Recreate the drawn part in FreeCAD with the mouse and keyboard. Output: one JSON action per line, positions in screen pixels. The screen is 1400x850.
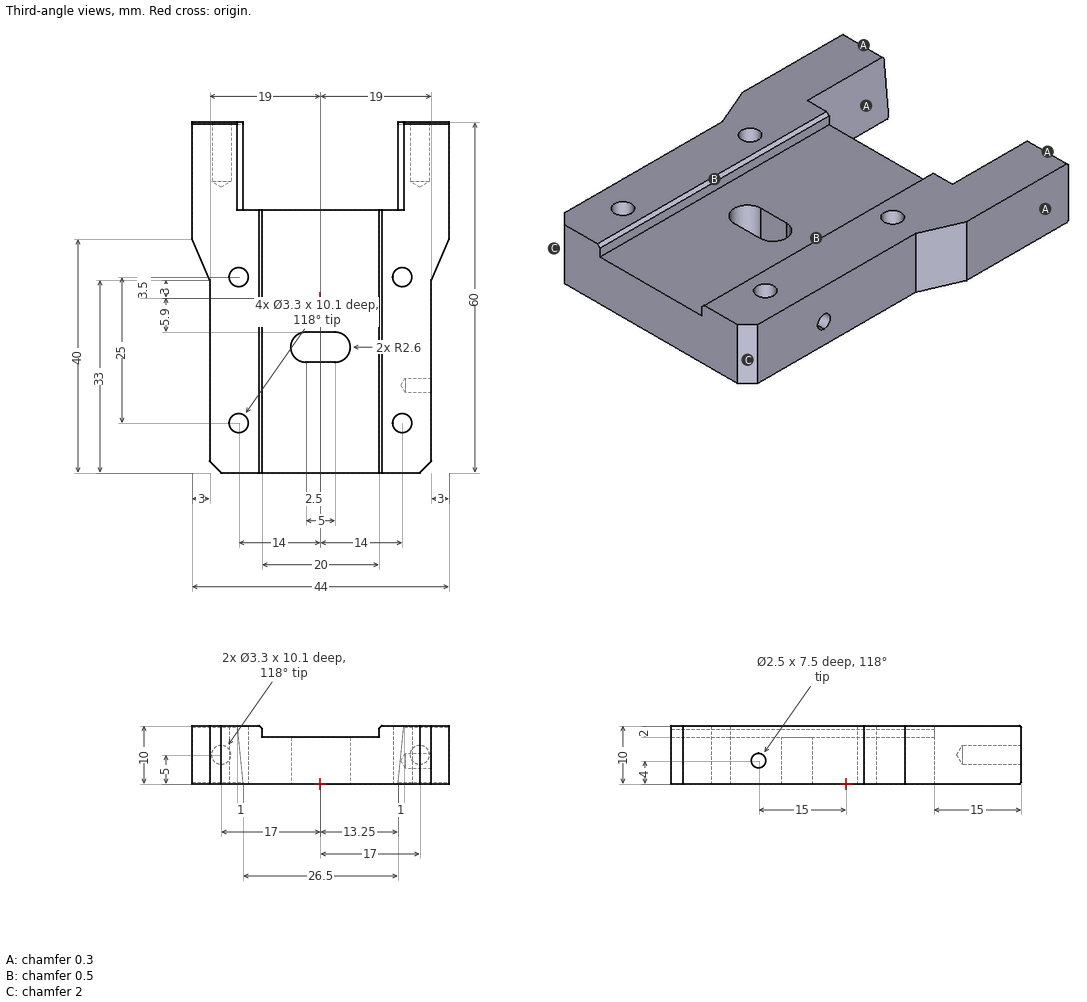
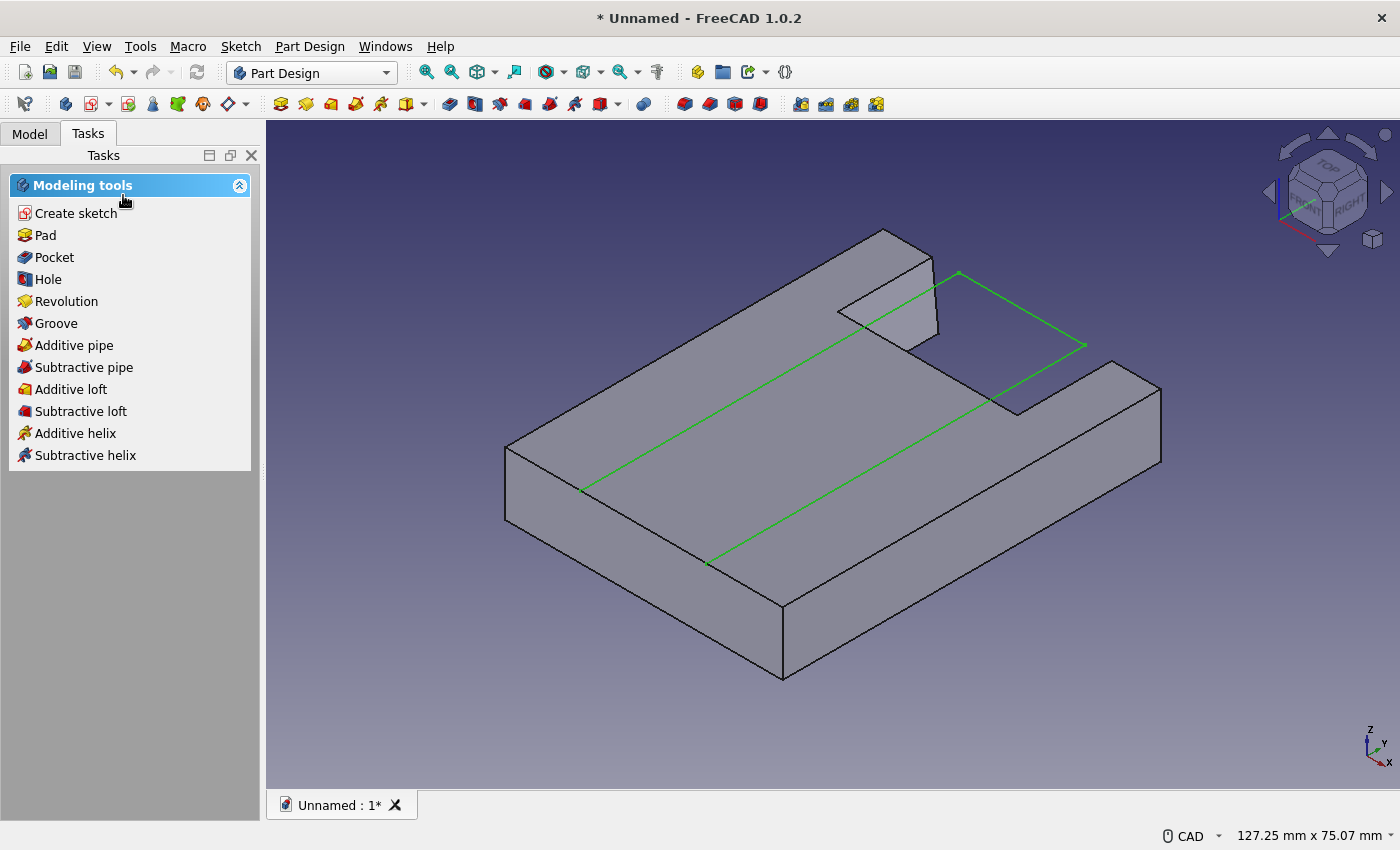
{"action": "left_click", "coordinate": [450, 104]}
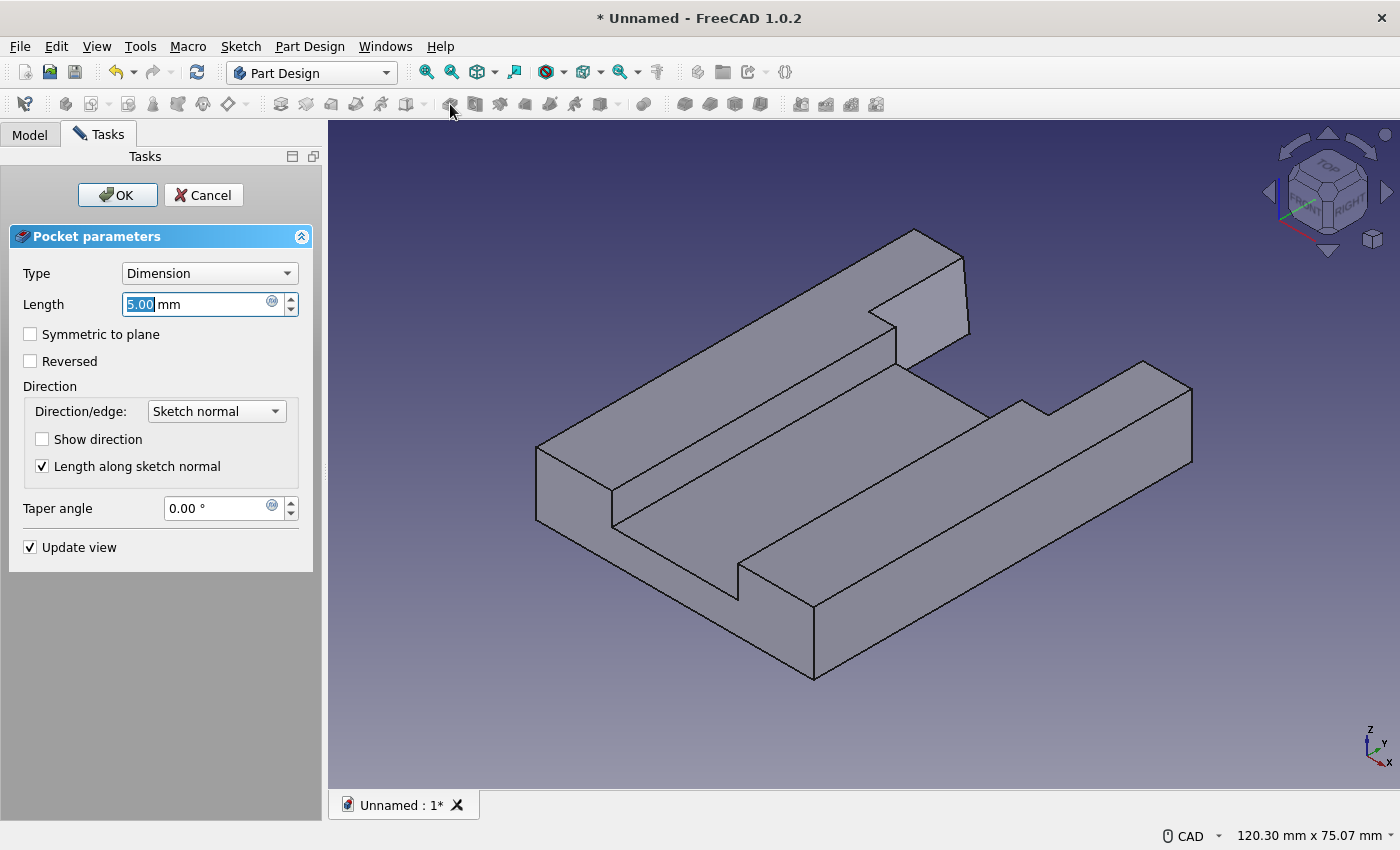
{"action": "type", "text": "2"}
{"action": "key", "text": "Tab"}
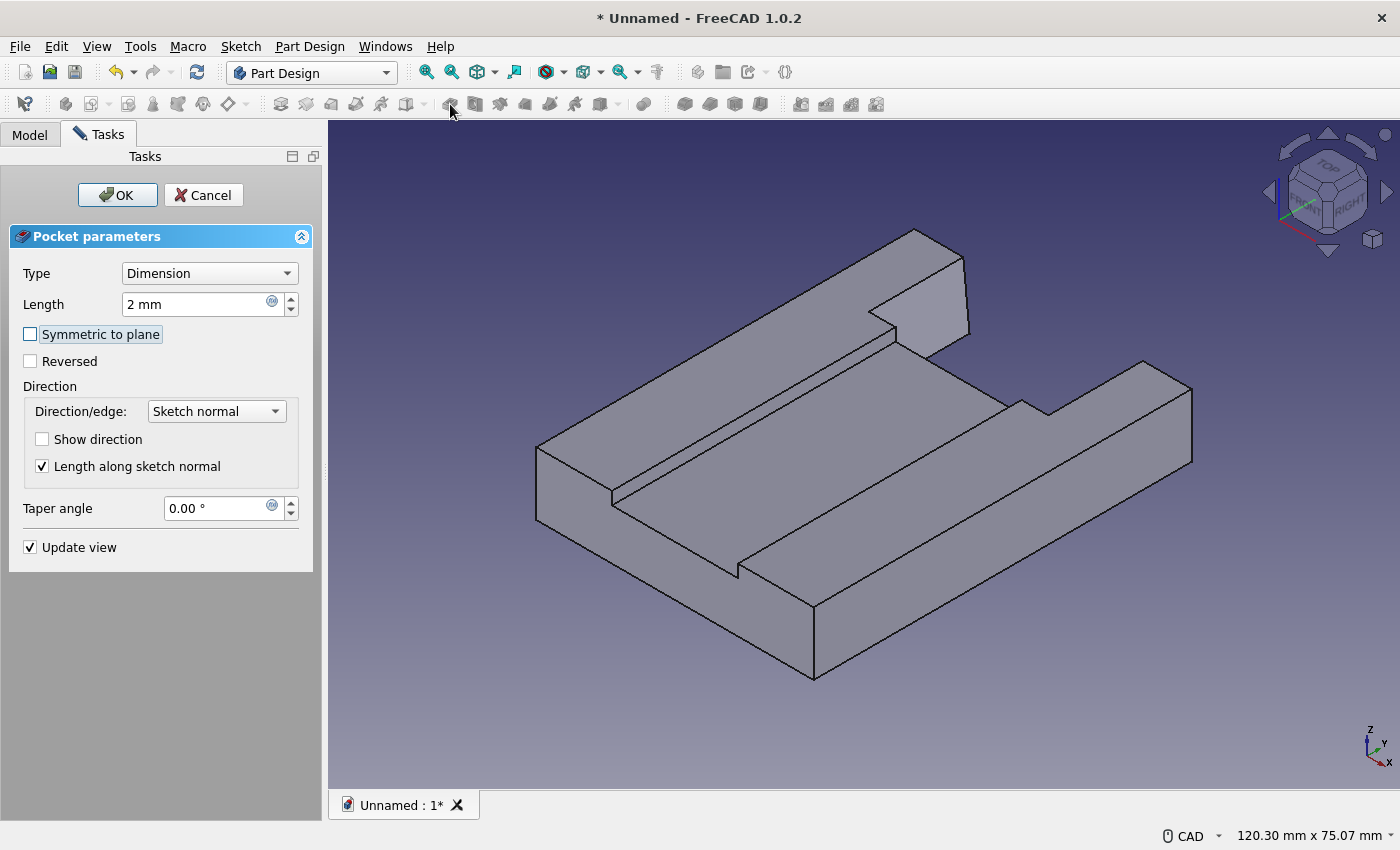
{"action": "left_click", "coordinate": [118, 195]}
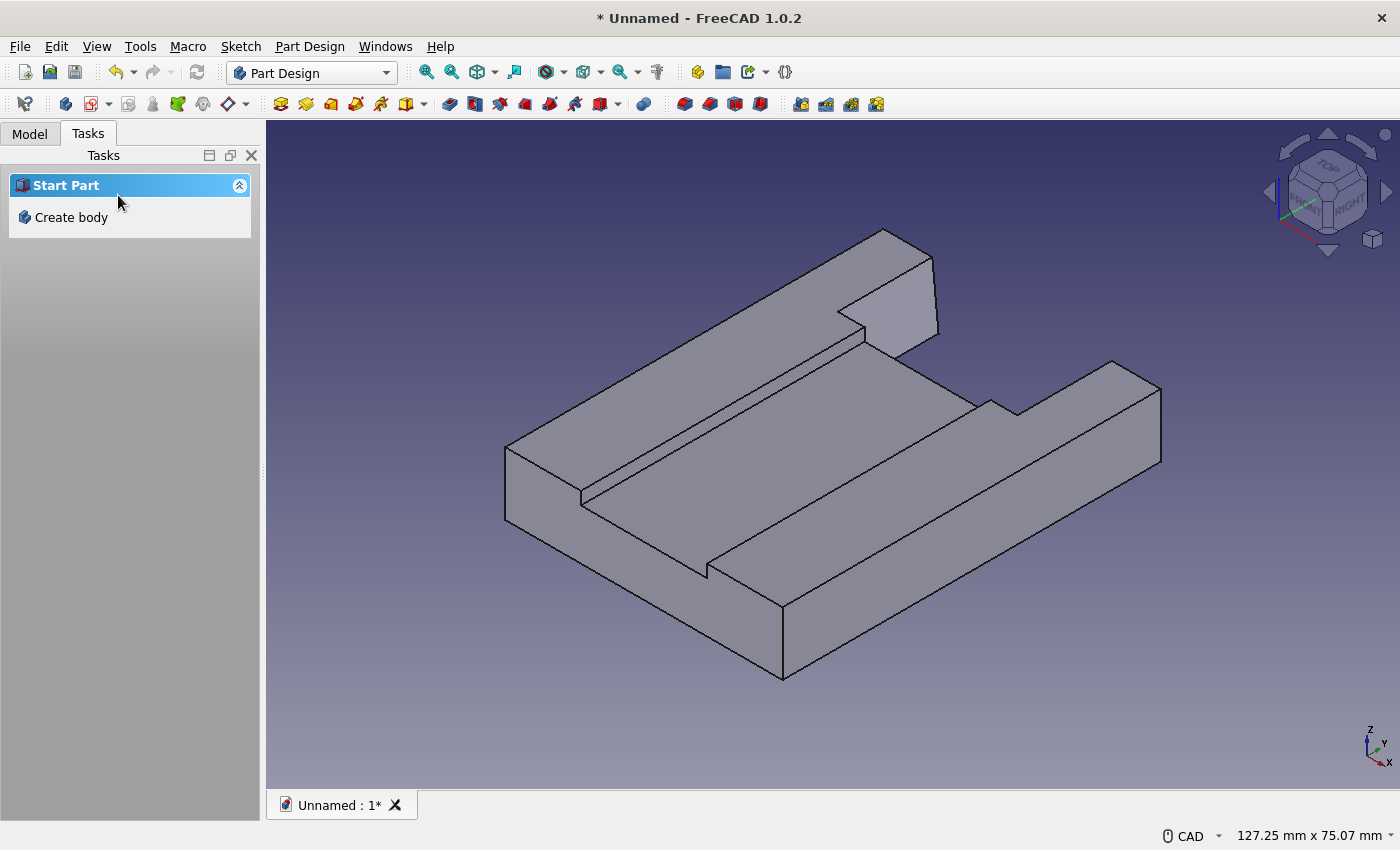
{"action": "key", "text": "4"}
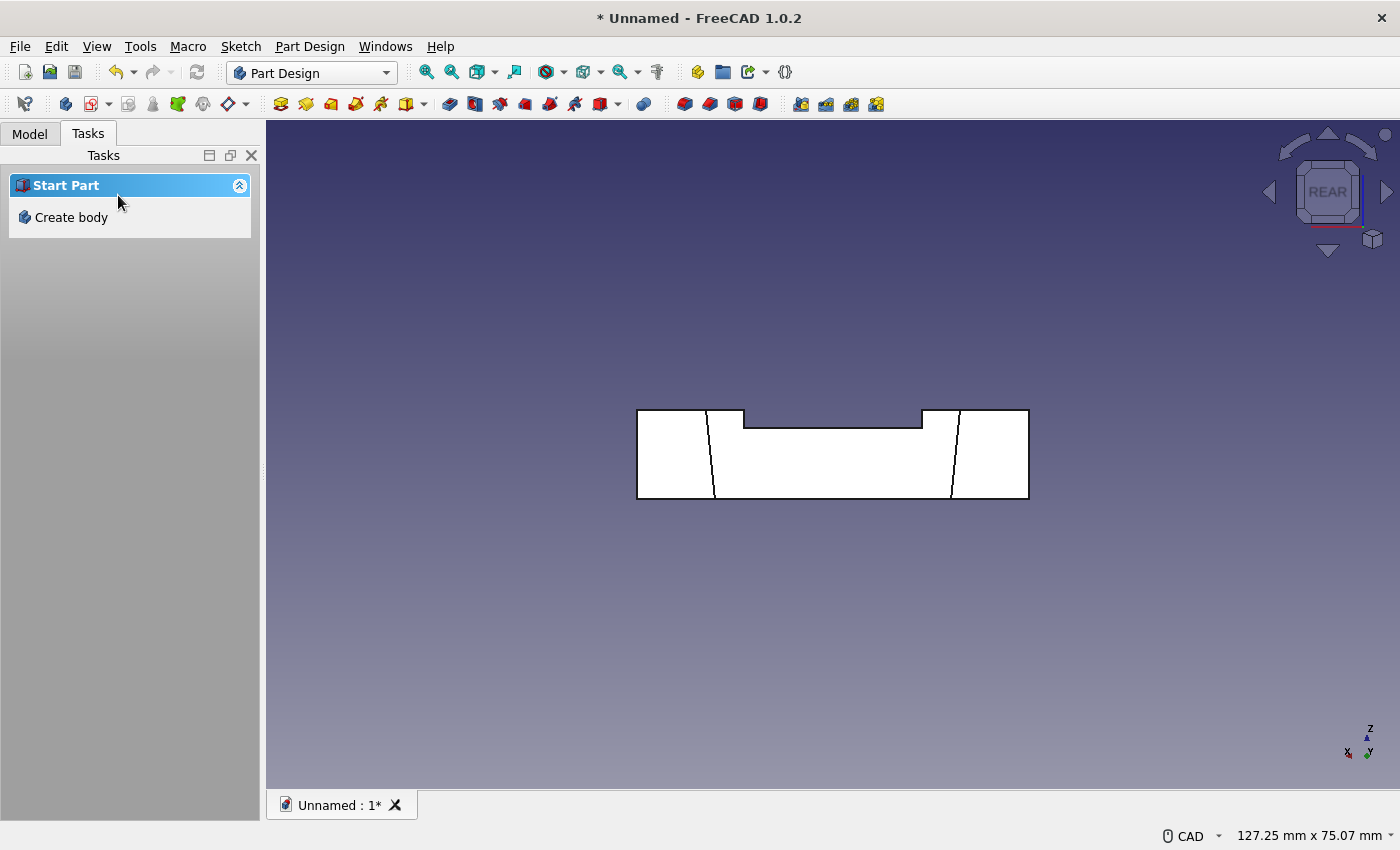
{"action": "left_click", "coordinate": [427, 72]}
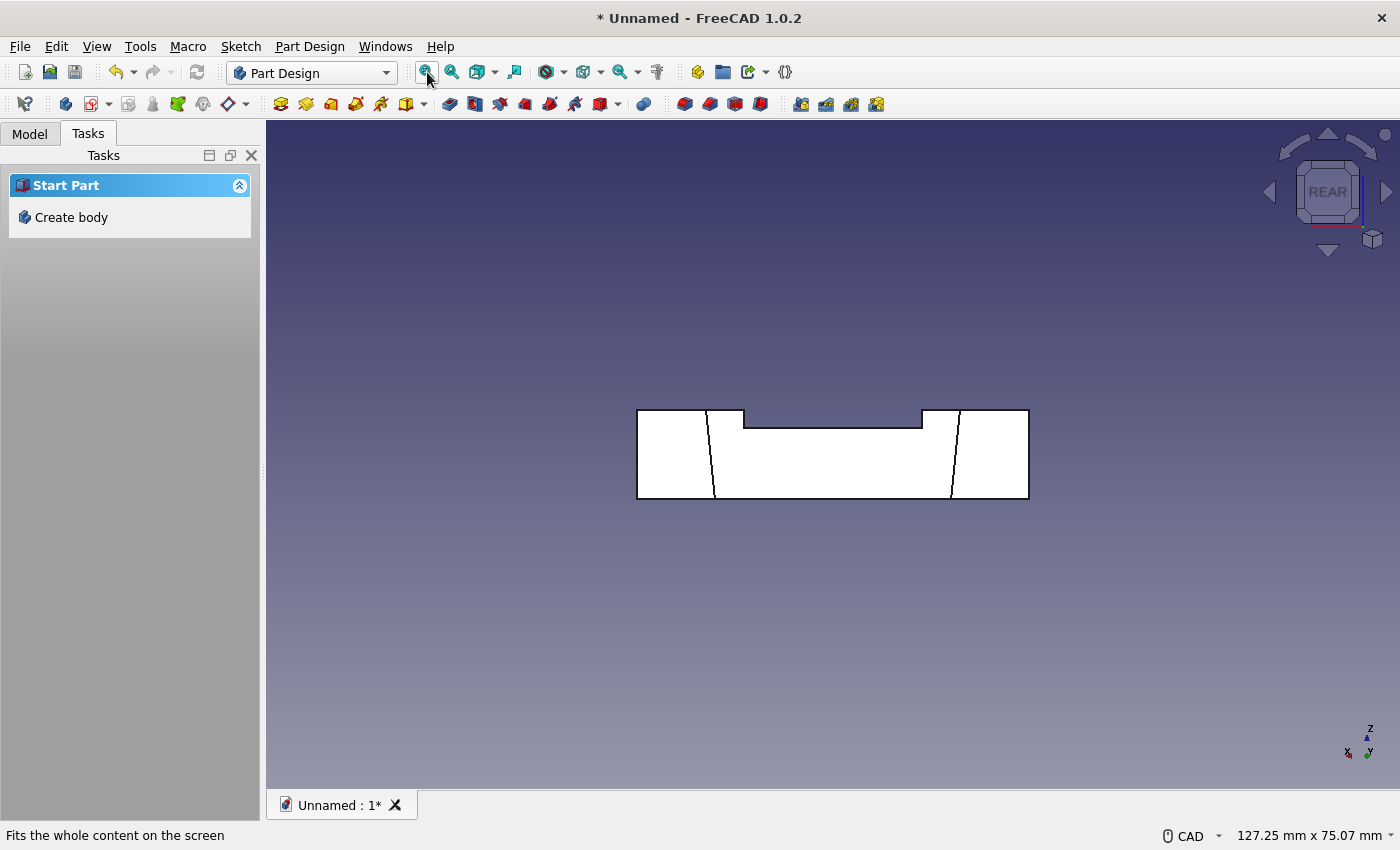
{"action": "left_click", "coordinate": [676, 454]}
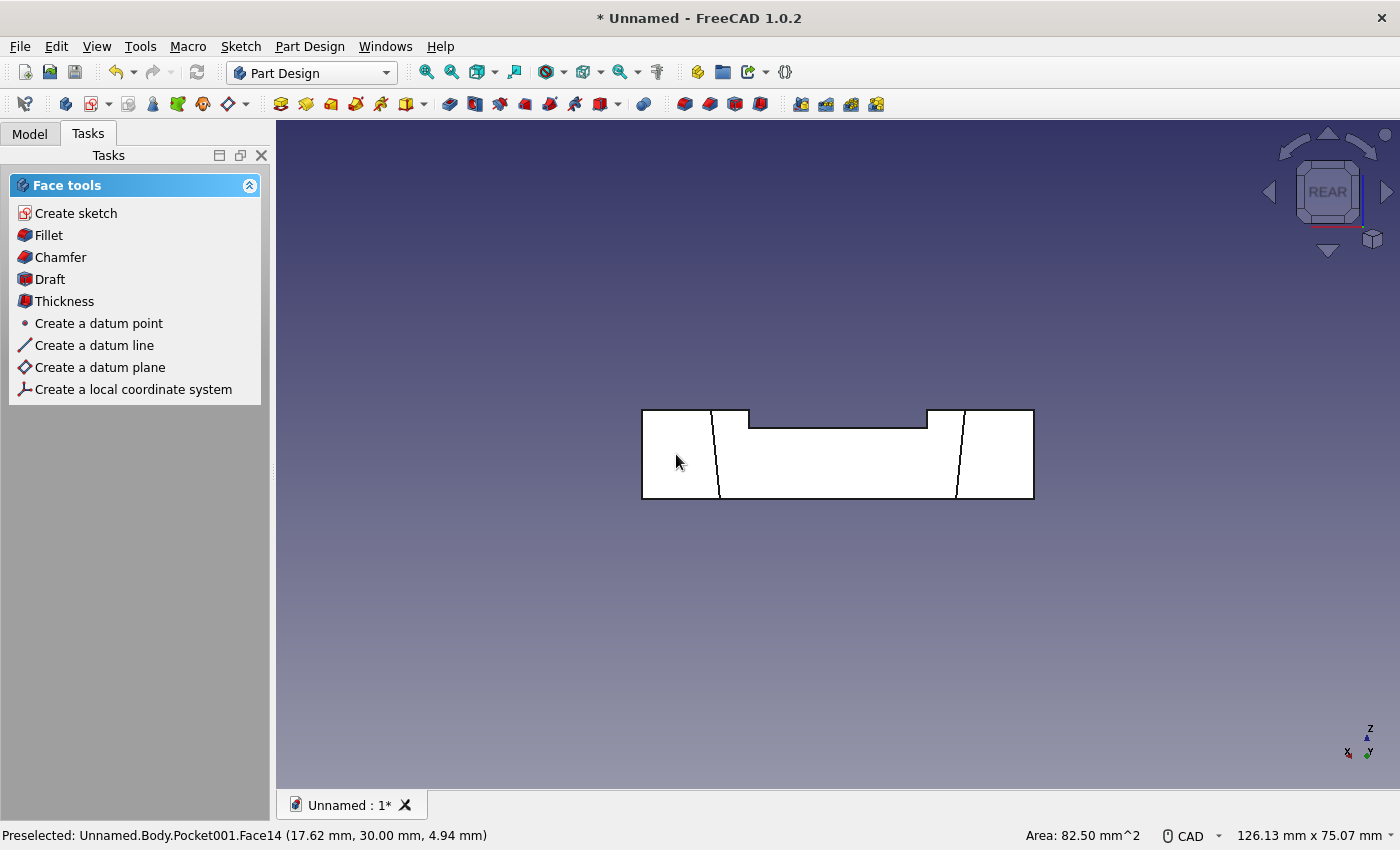
{"action": "left_click", "coordinate": [90, 104]}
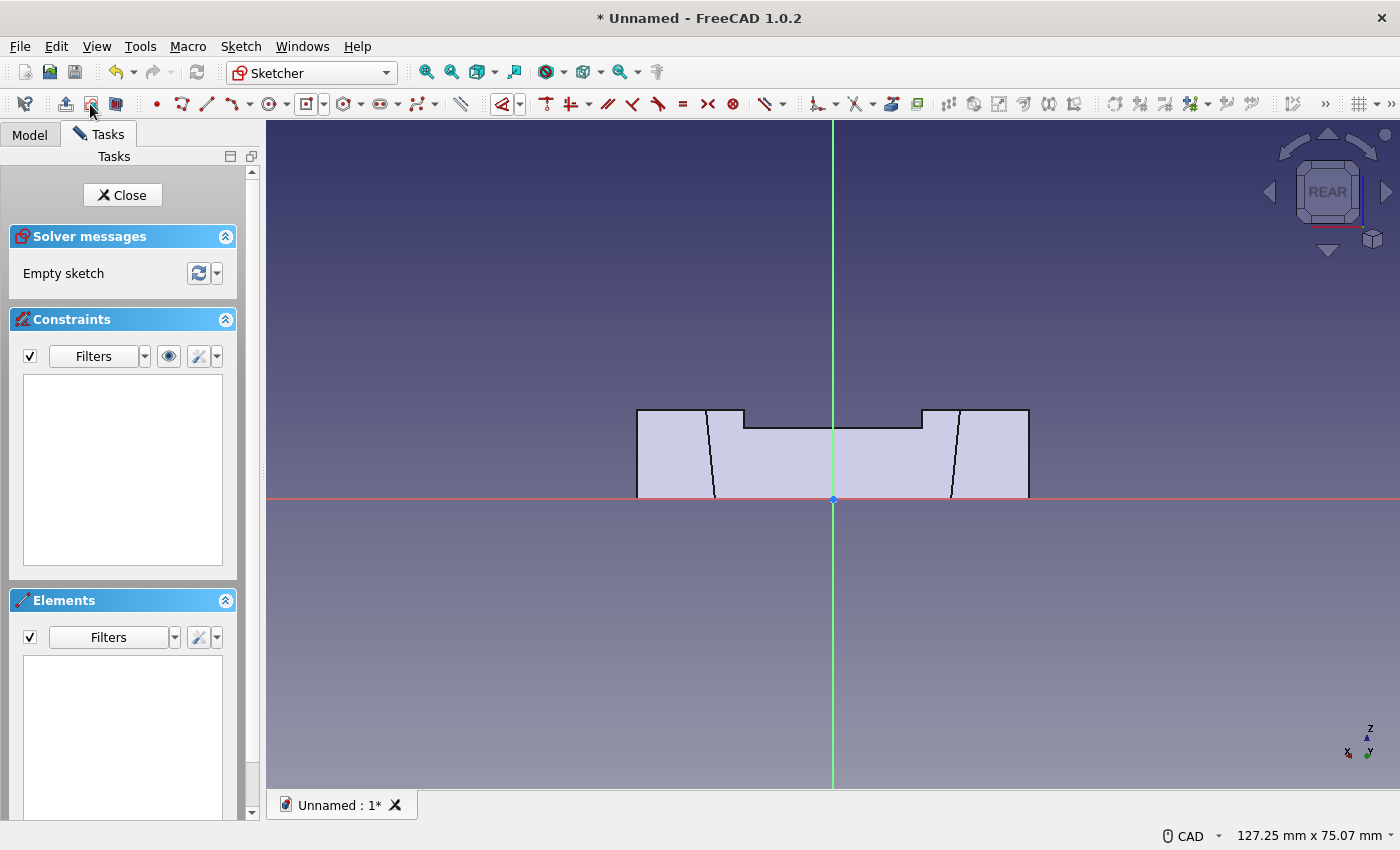
{"action": "scroll", "coordinate": [916, 488], "scroll_direction": "up", "scroll_amount": 3}